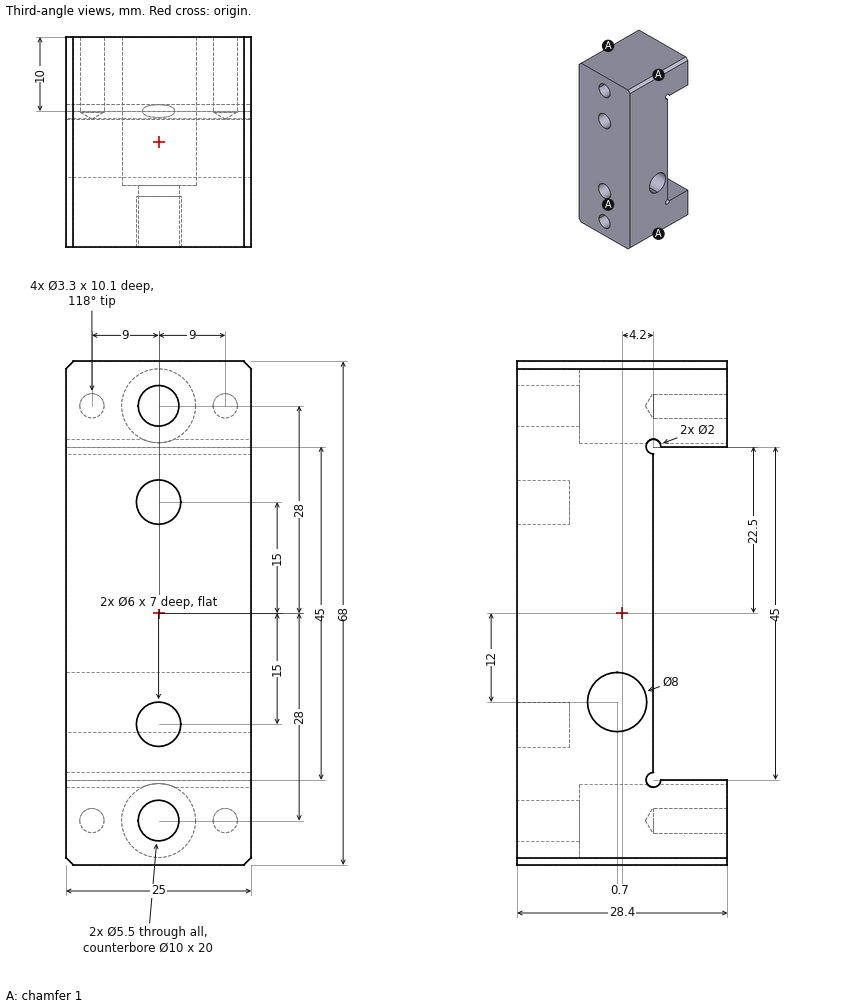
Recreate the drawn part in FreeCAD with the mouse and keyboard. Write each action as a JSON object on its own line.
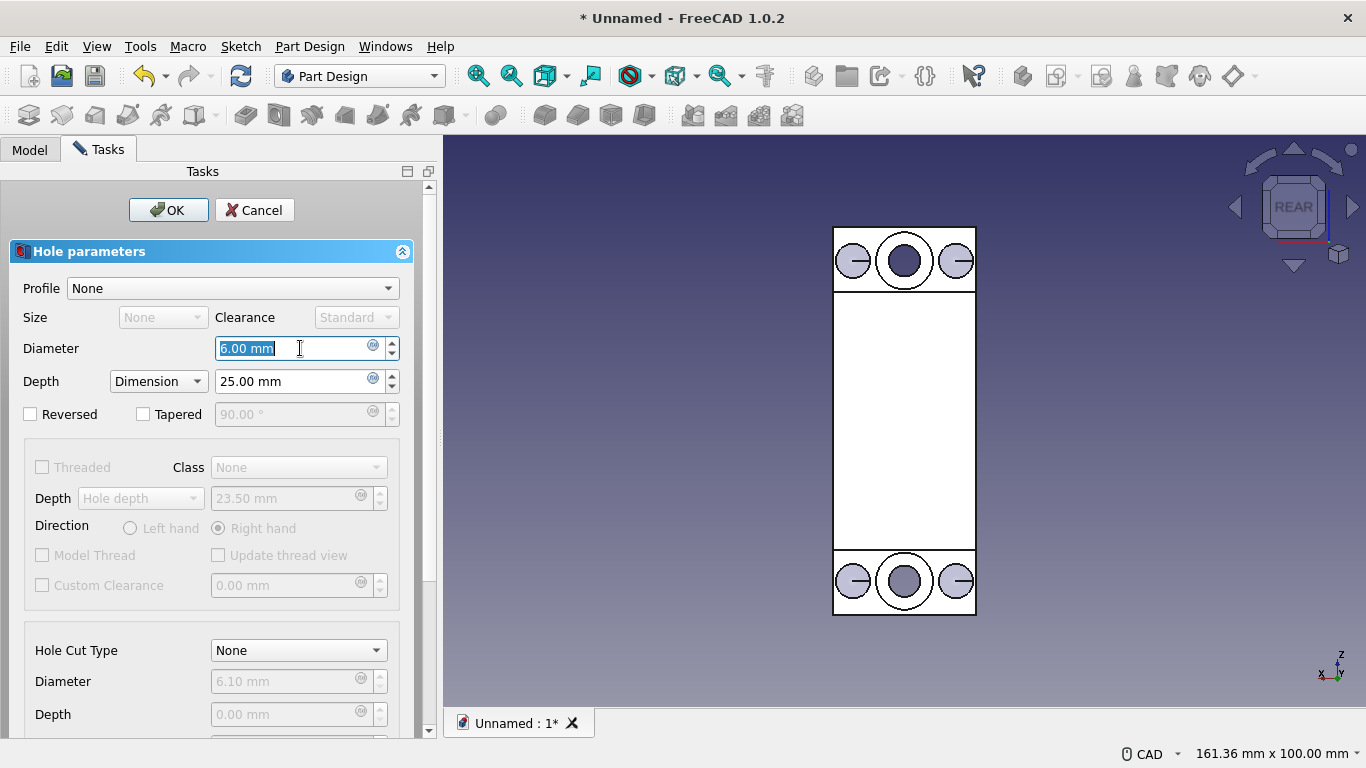
{"action": "type", "text": "3.3"}
{"action": "key", "text": "Tab"}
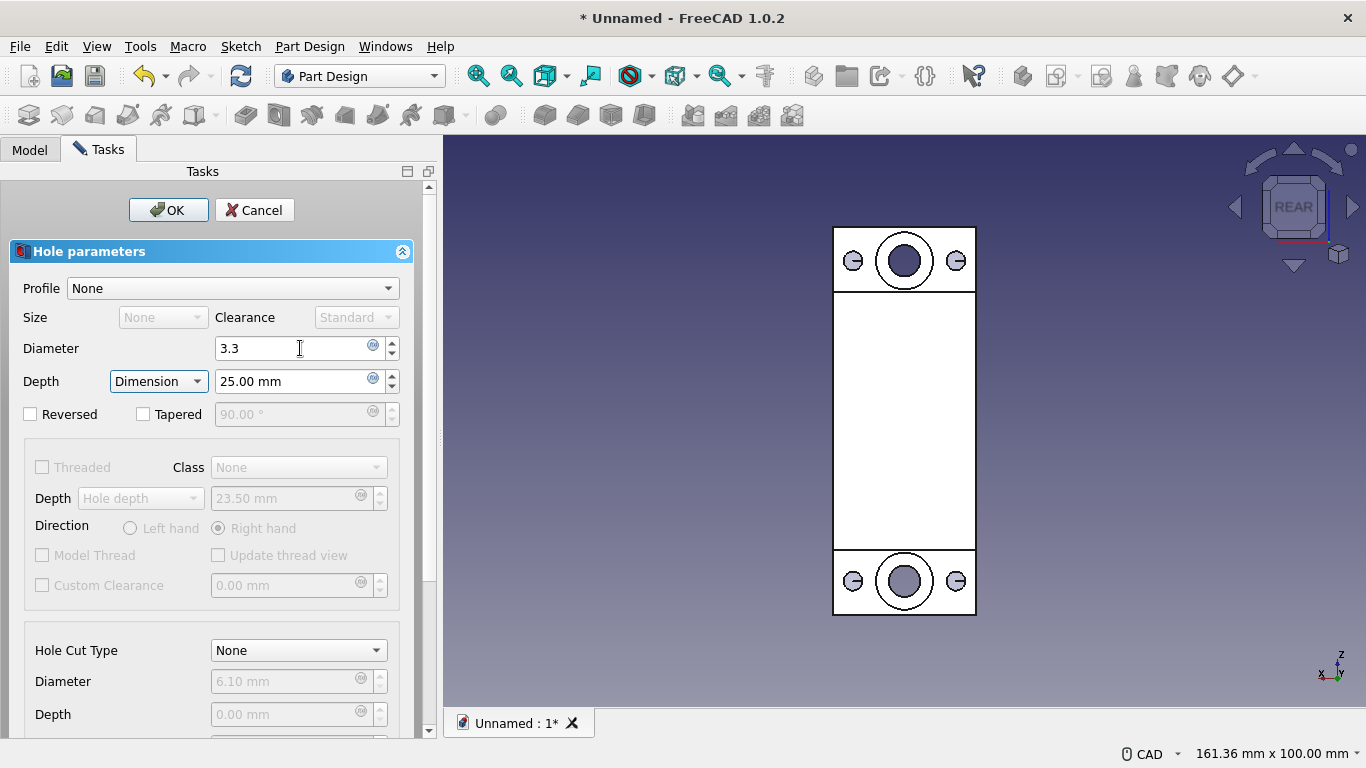
{"action": "triple_click", "coordinate": [300, 382]}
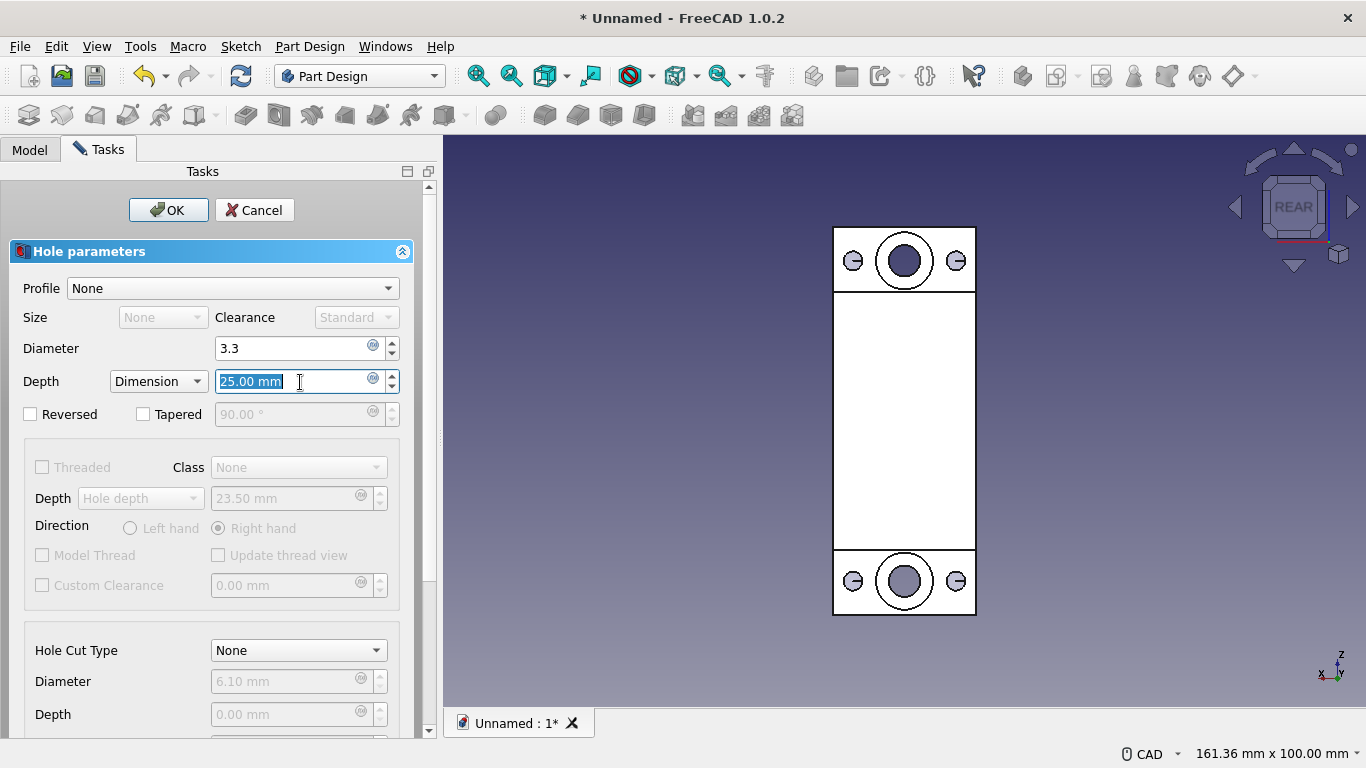
{"action": "type", "text": "10.1"}
{"action": "key", "text": "Tab"}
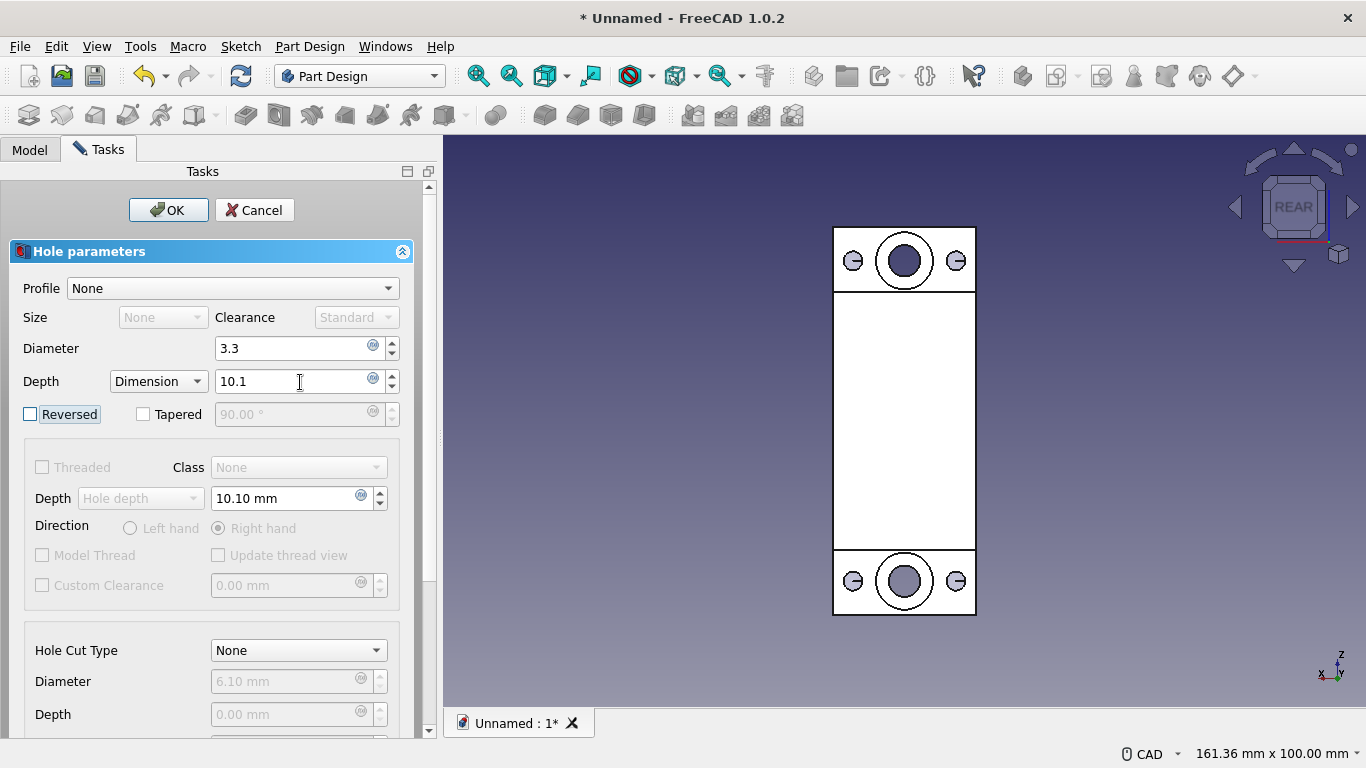
{"action": "left_click", "coordinate": [169, 210]}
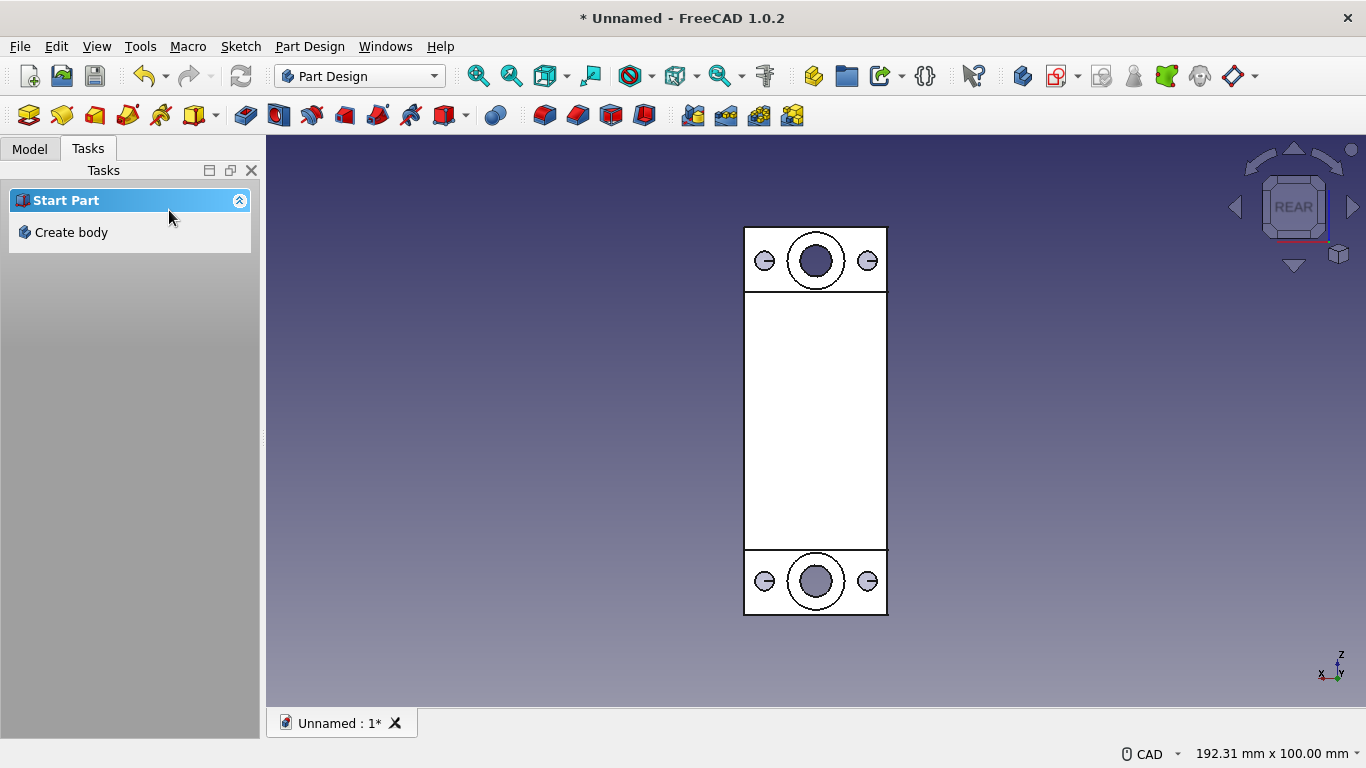
{"action": "key", "text": "0"}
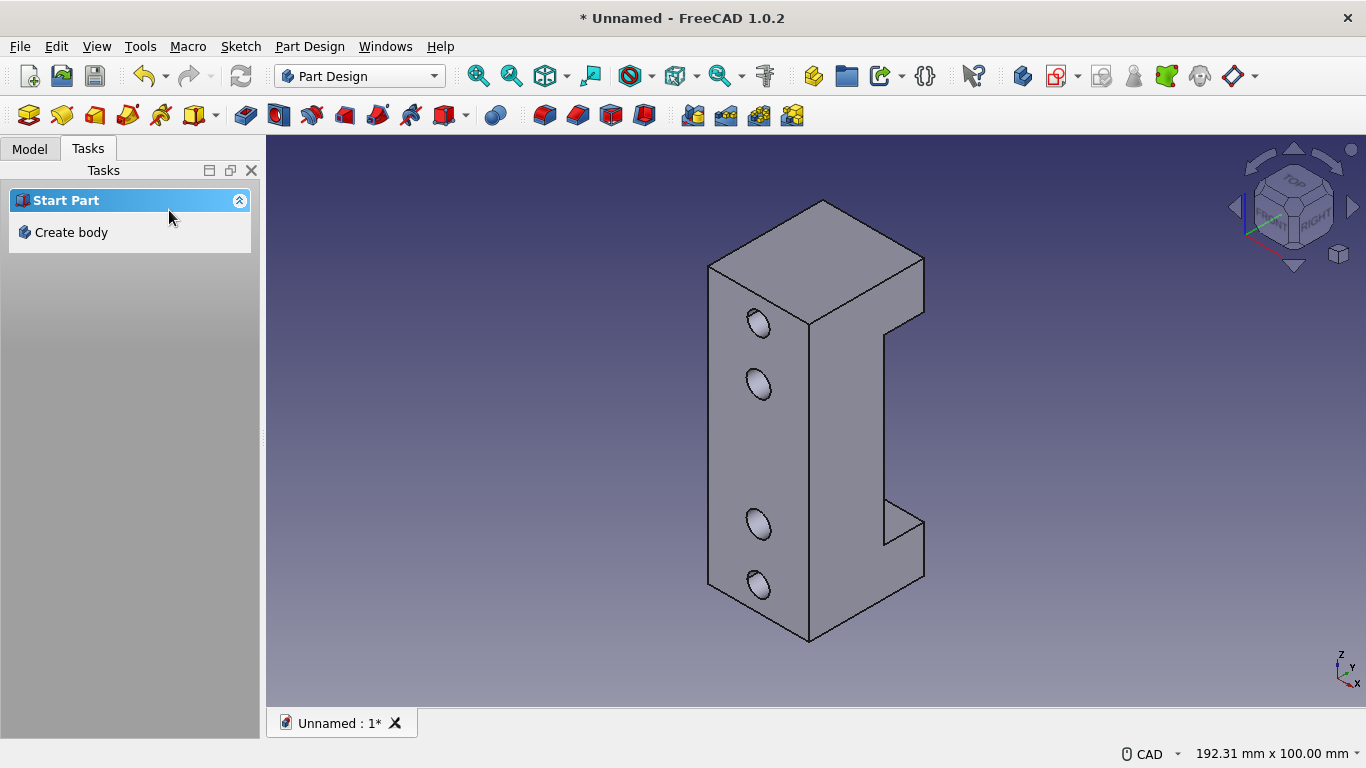
{"action": "left_click", "coordinate": [867, 290]}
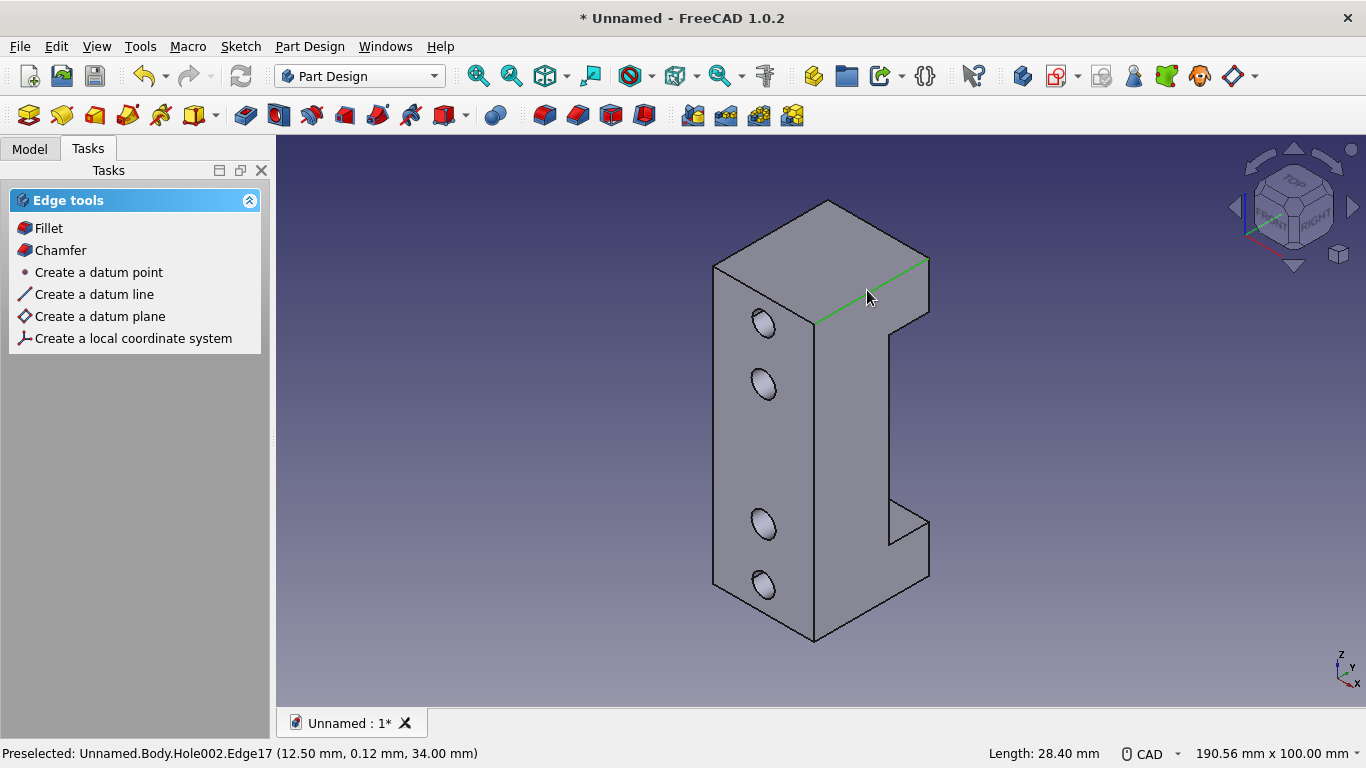
{"action": "key", "text": "2"}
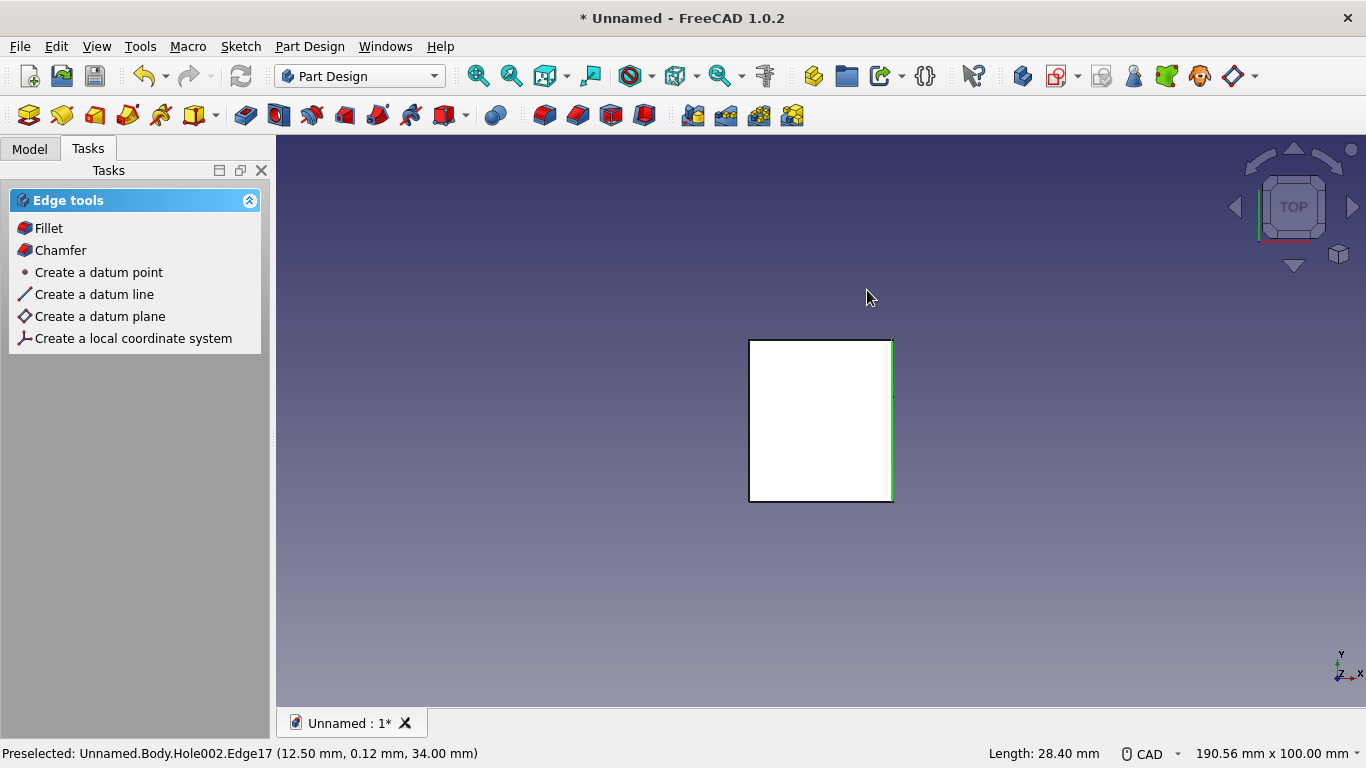
{"action": "key", "text": "v f"}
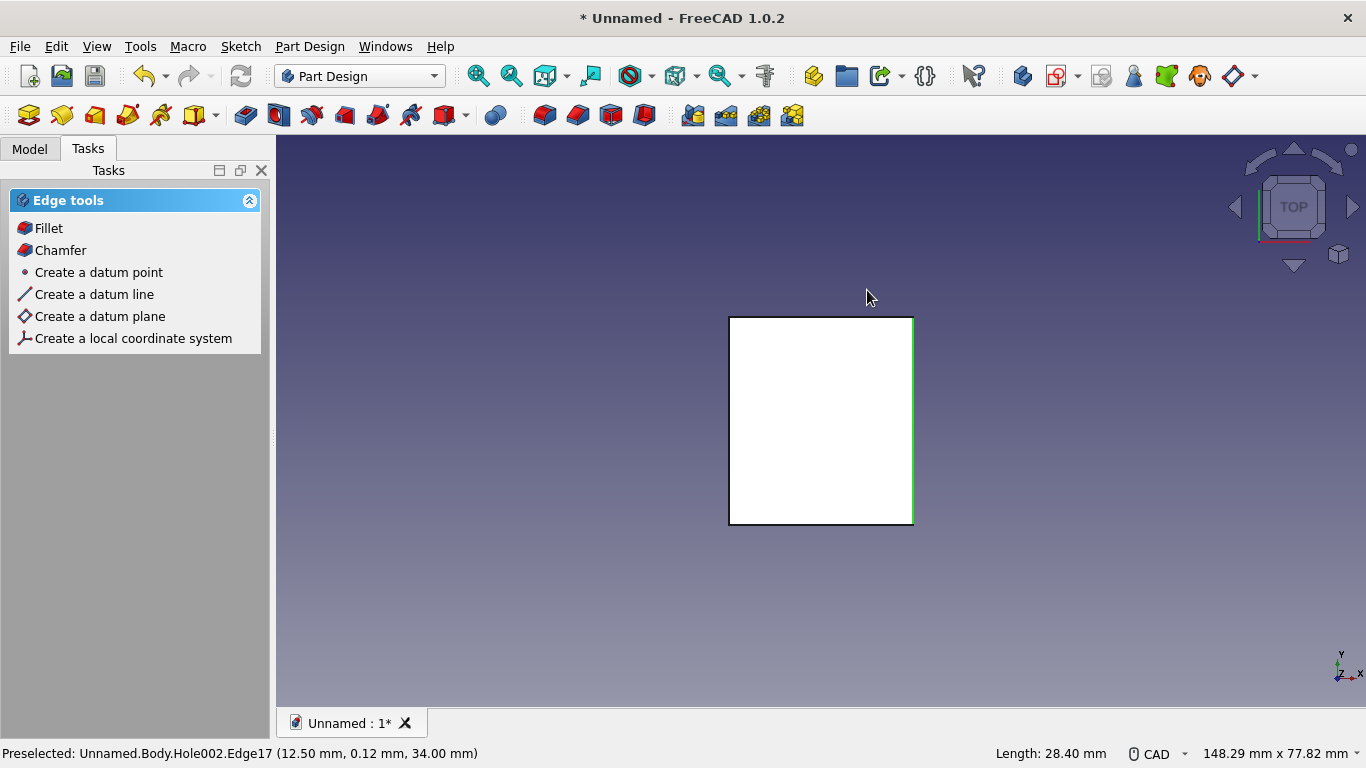
{"action": "left_click", "coordinate": [729, 420], "text": "ctrl"}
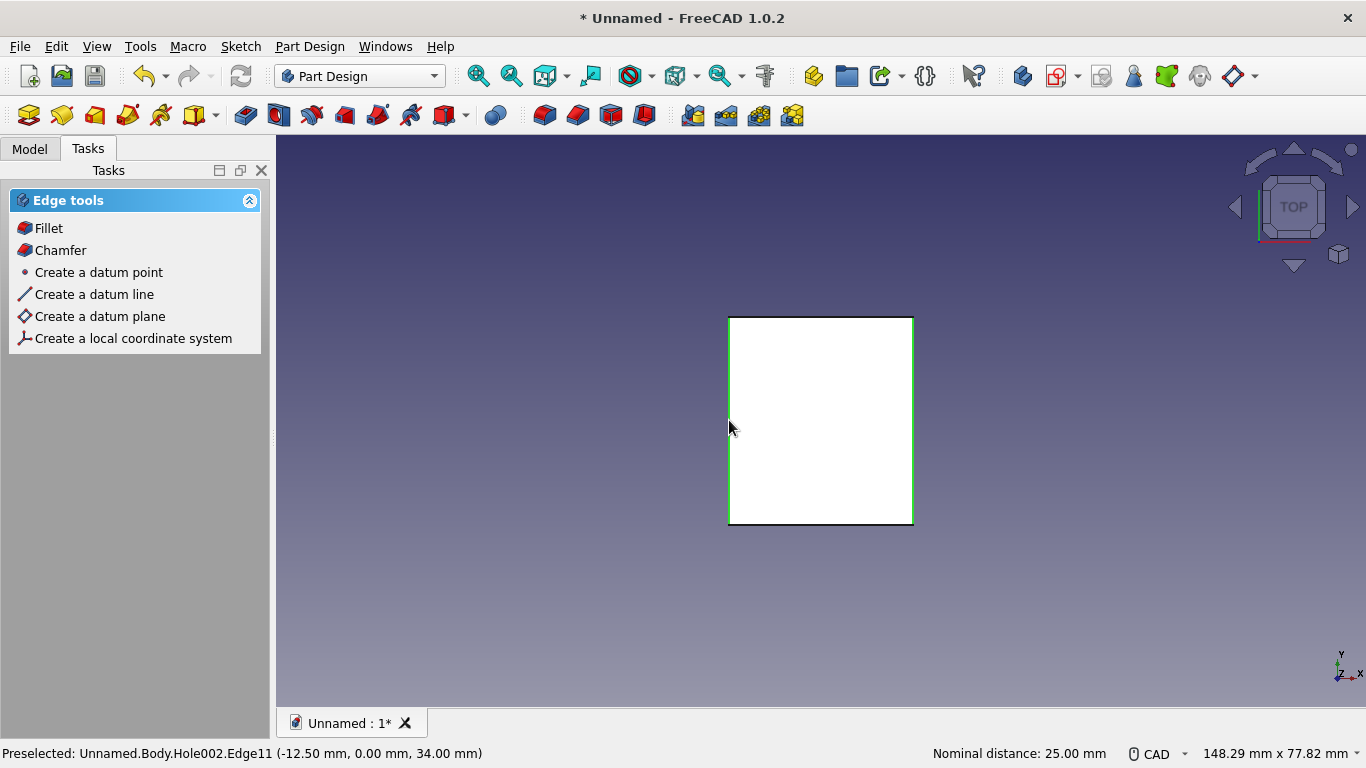
{"action": "key", "text": "1"}